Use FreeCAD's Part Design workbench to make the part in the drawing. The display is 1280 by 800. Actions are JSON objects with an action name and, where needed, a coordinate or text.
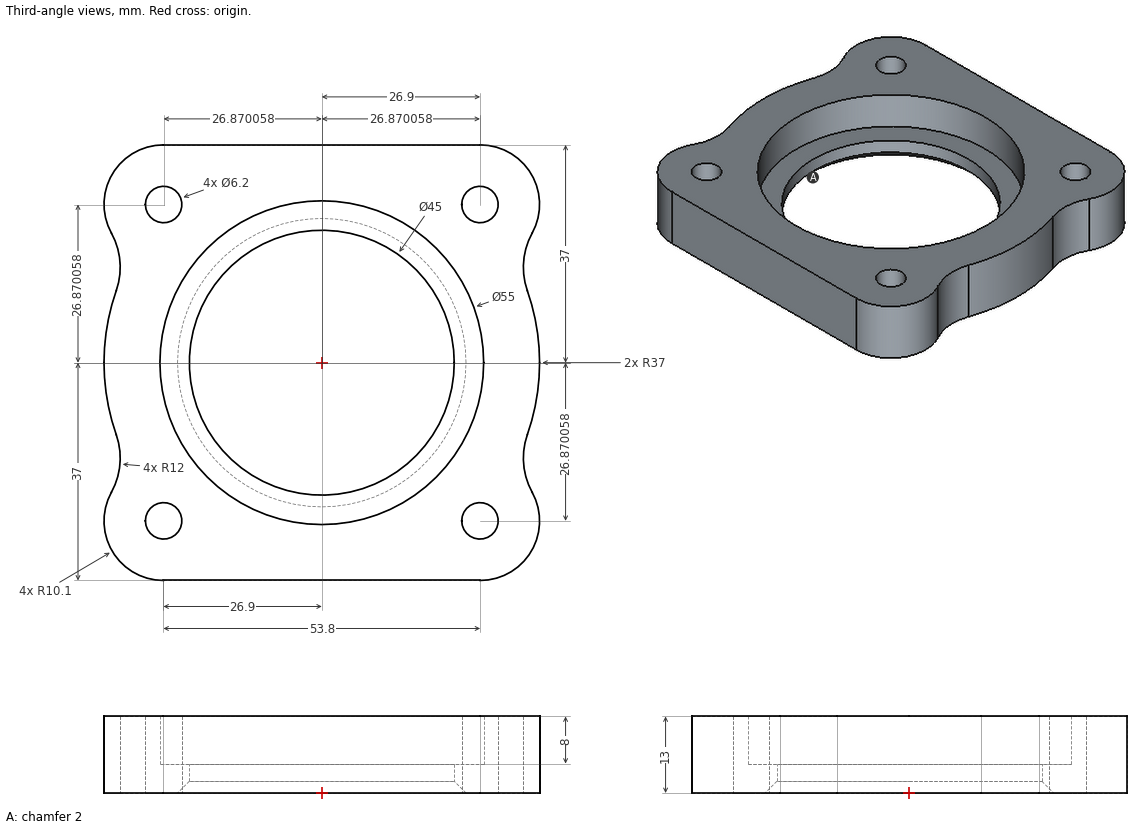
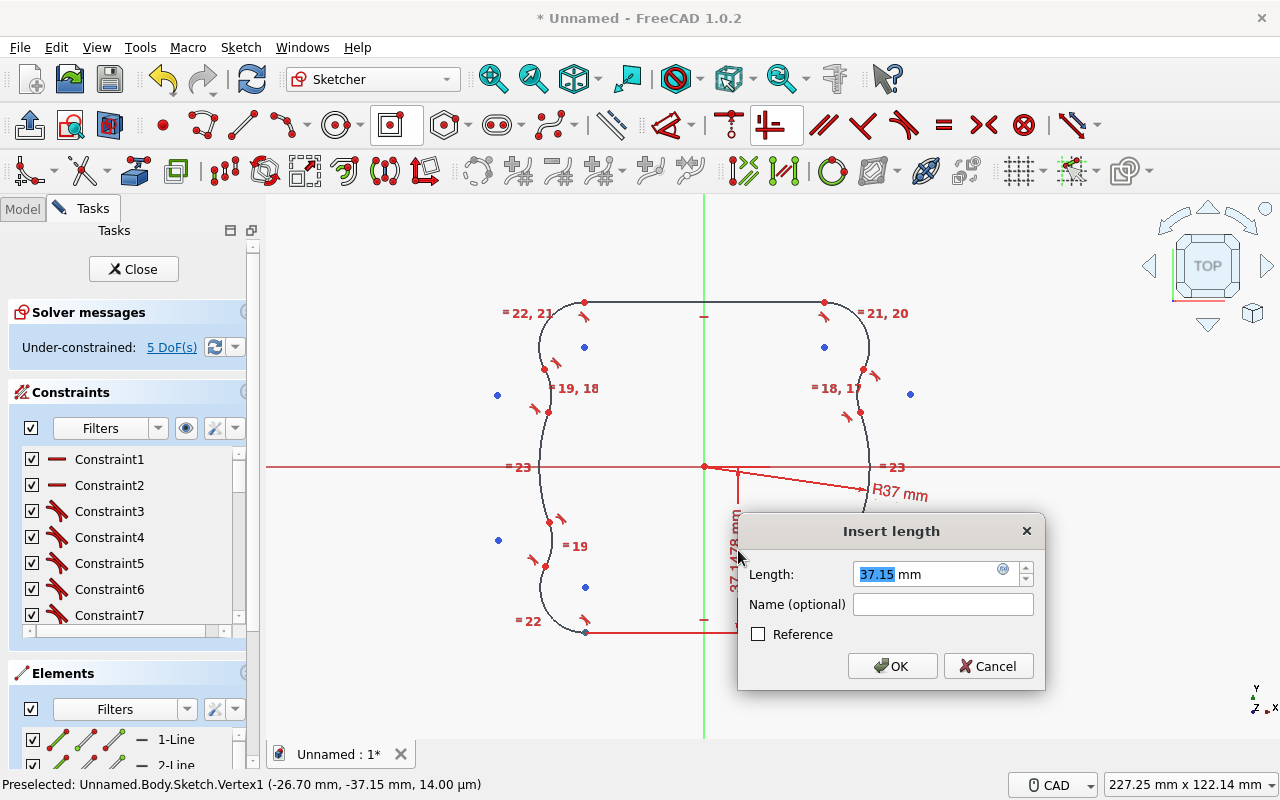
{"action": "type", "text": "37"}
{"action": "key", "text": "Return"}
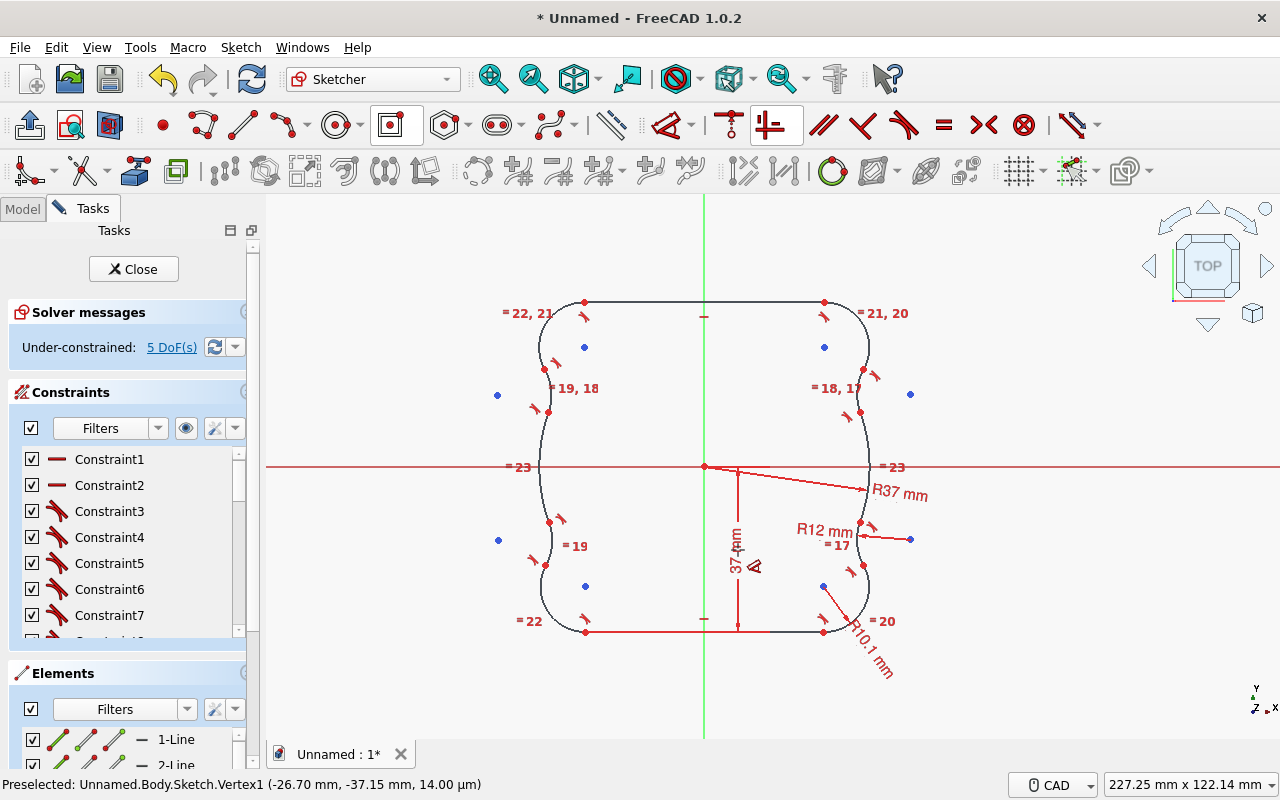
{"action": "left_click", "coordinate": [824, 302]}
{"action": "left_click", "coordinate": [670, 385]}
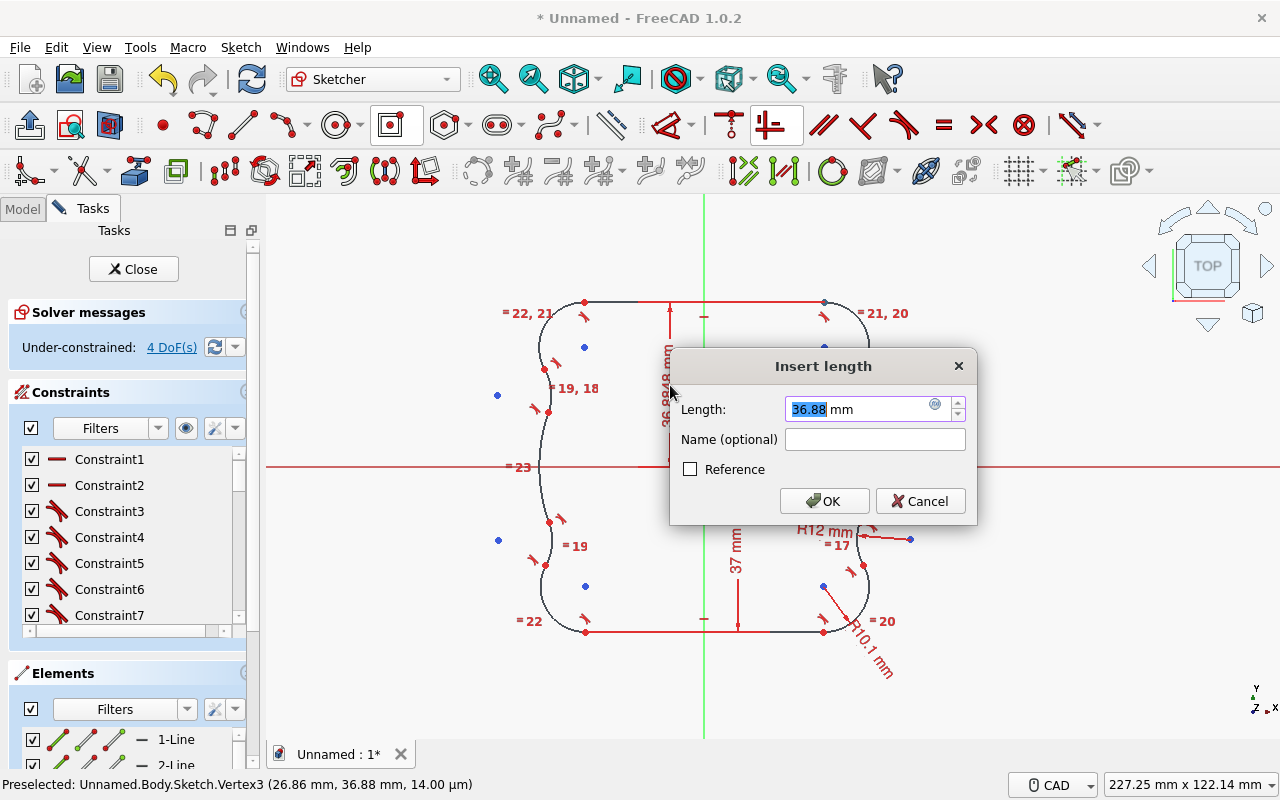
{"action": "type", "text": "37"}
{"action": "key", "text": "Return"}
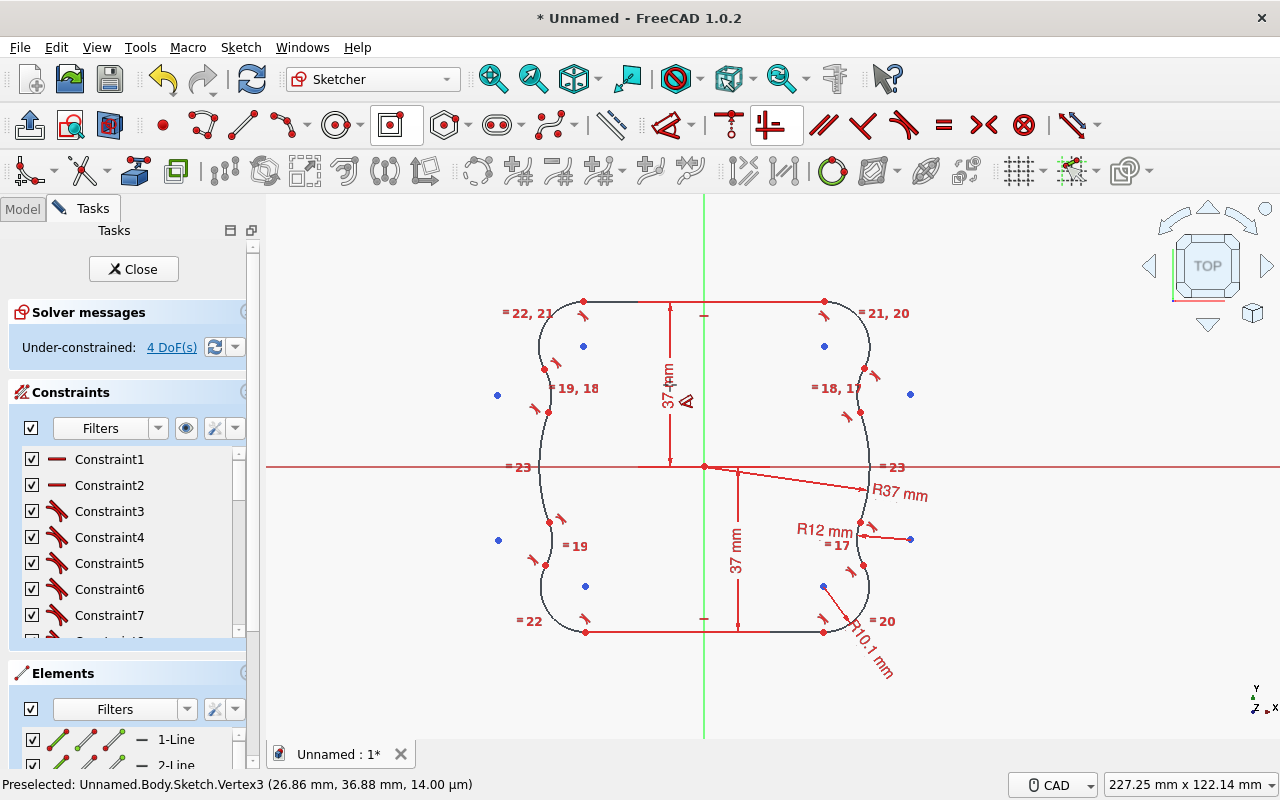
{"action": "left_click", "coordinate": [657, 632]}
{"action": "left_click", "coordinate": [650, 666]}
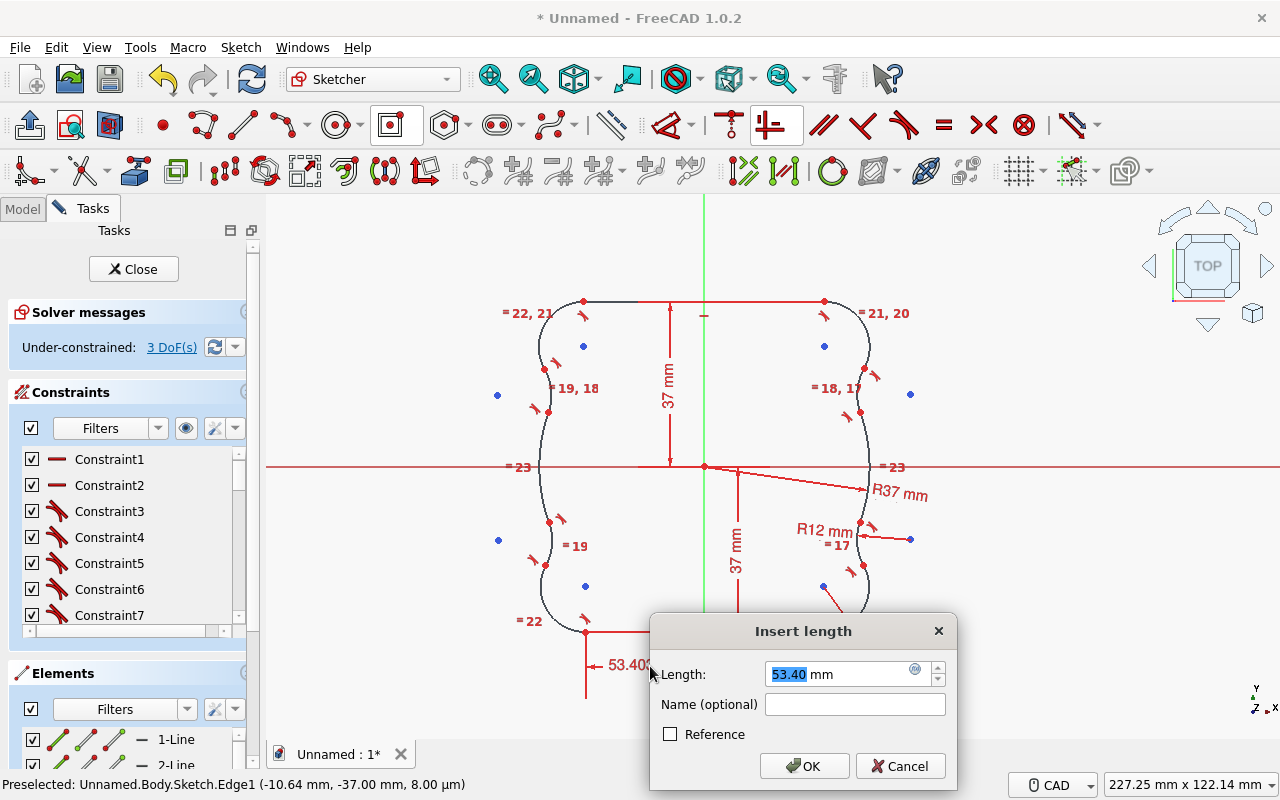
{"action": "type", "text": "53.8"}
{"action": "key", "text": "Return"}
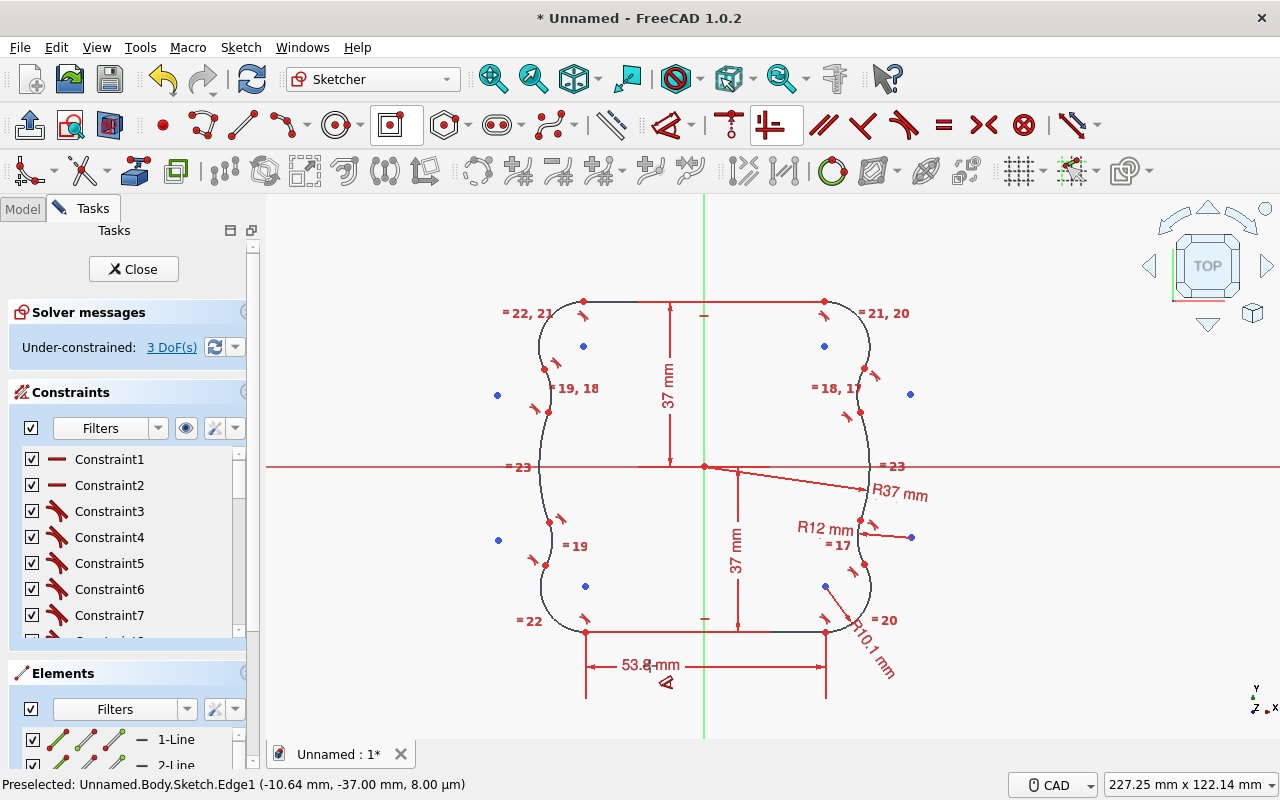
{"action": "left_click", "coordinate": [752, 302]}
{"action": "left_click", "coordinate": [649, 268]}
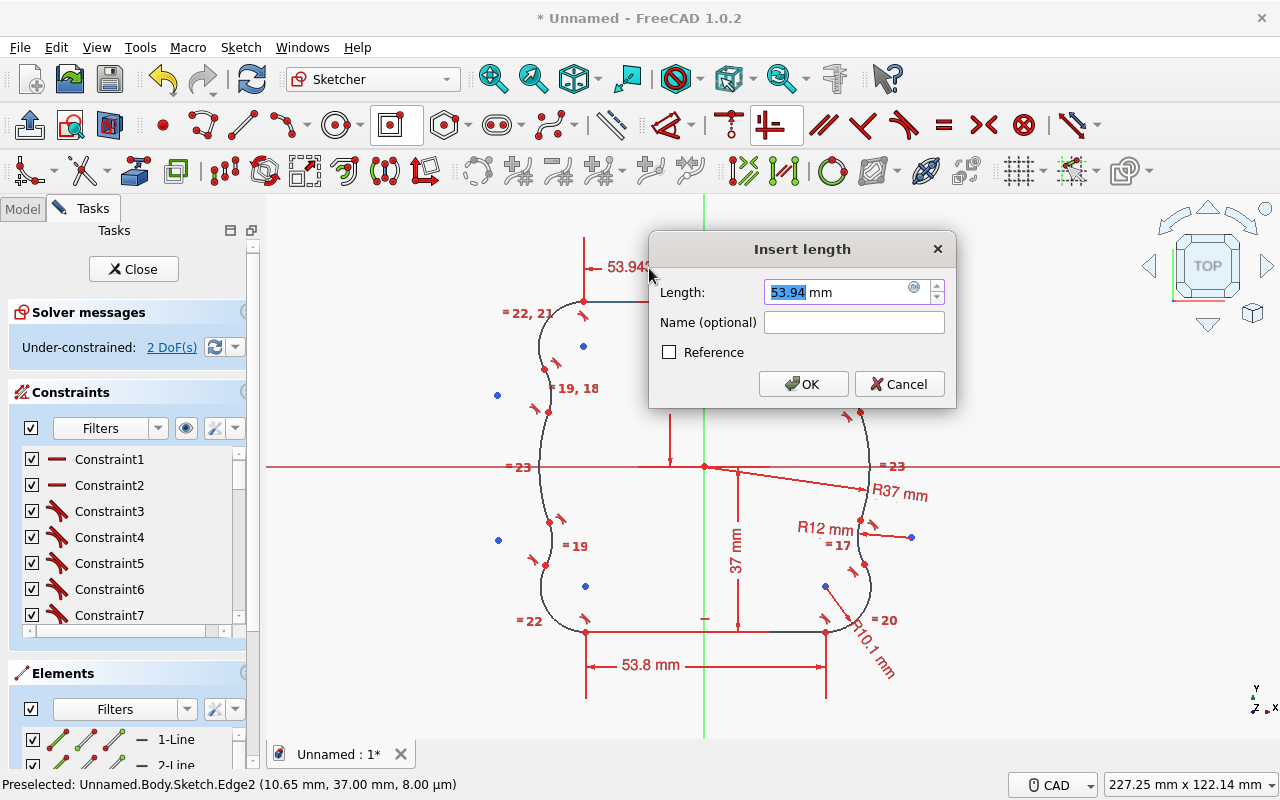
{"action": "type", "text": "53.8"}
{"action": "key", "text": "Return"}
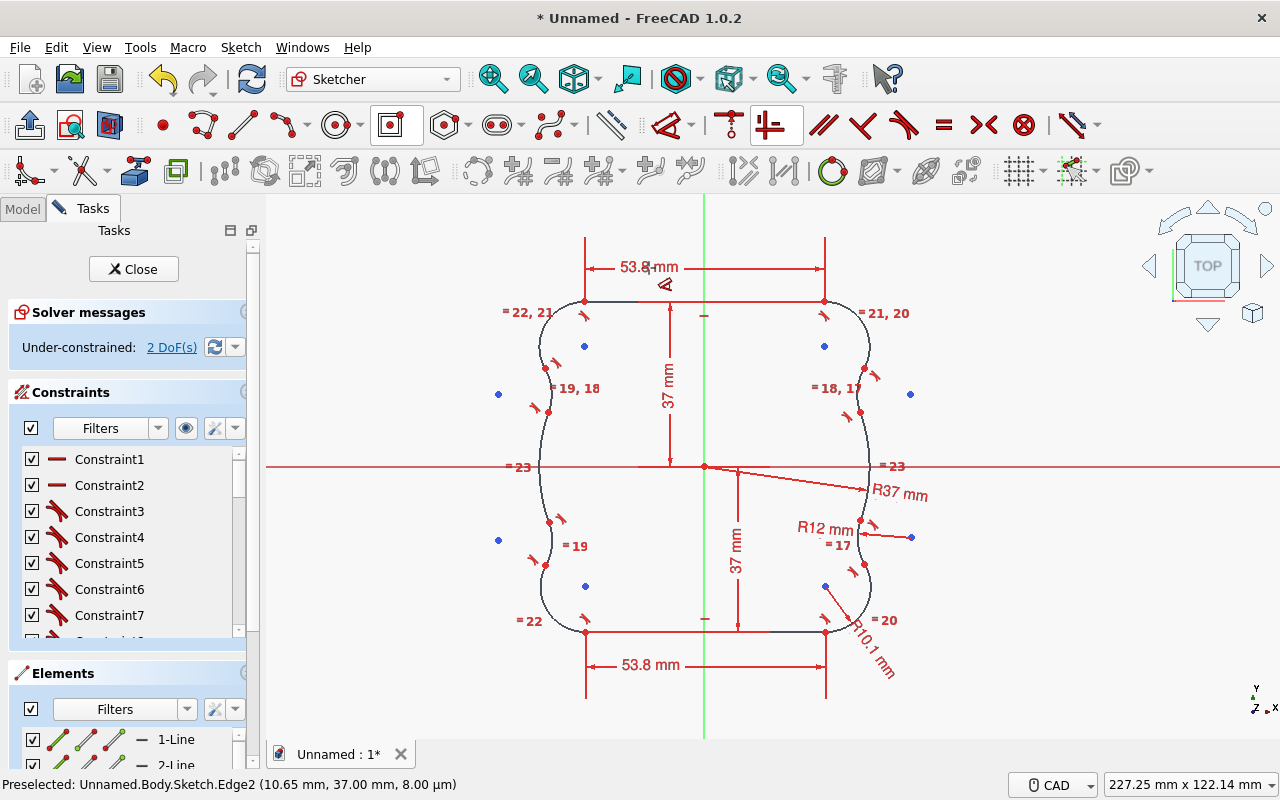
{"action": "left_click", "coordinate": [586, 632]}
{"action": "left_click", "coordinate": [645, 433]}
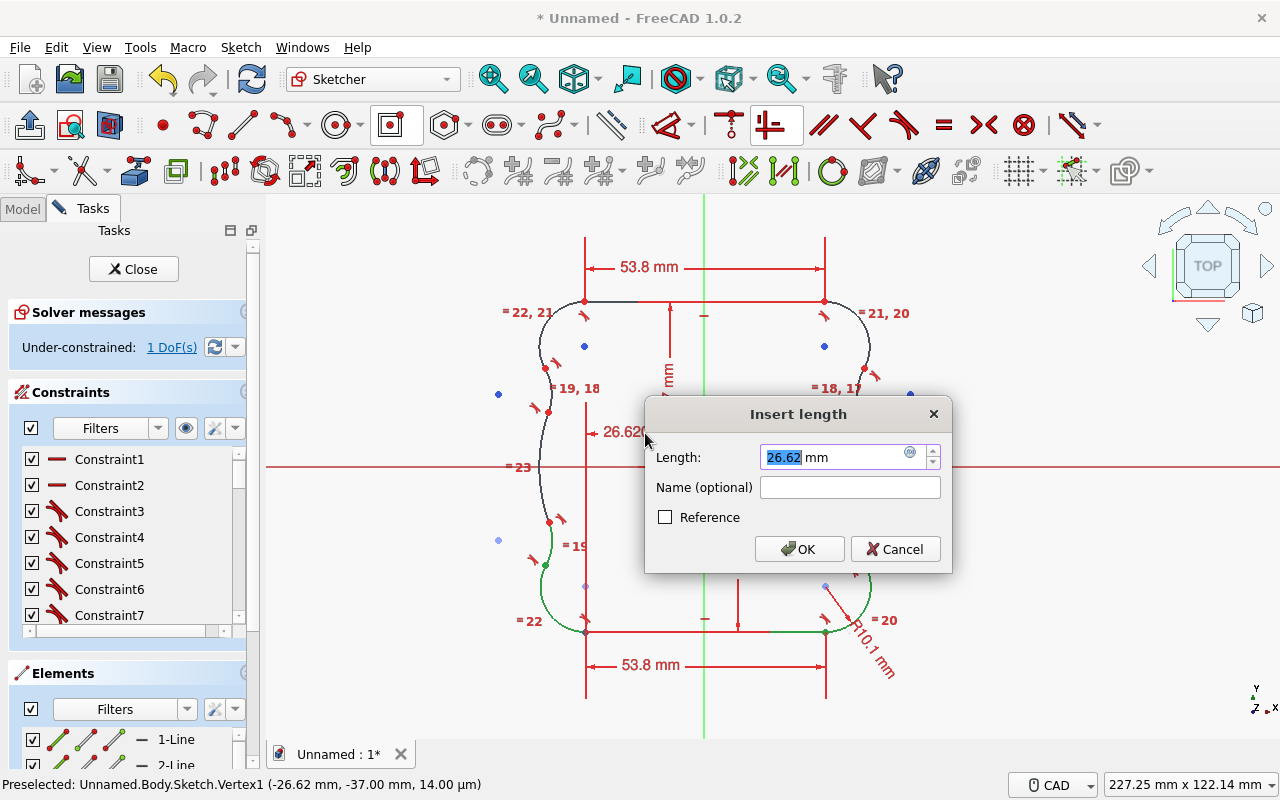
{"action": "type", "text": "26.9"}
{"action": "key", "text": "Return"}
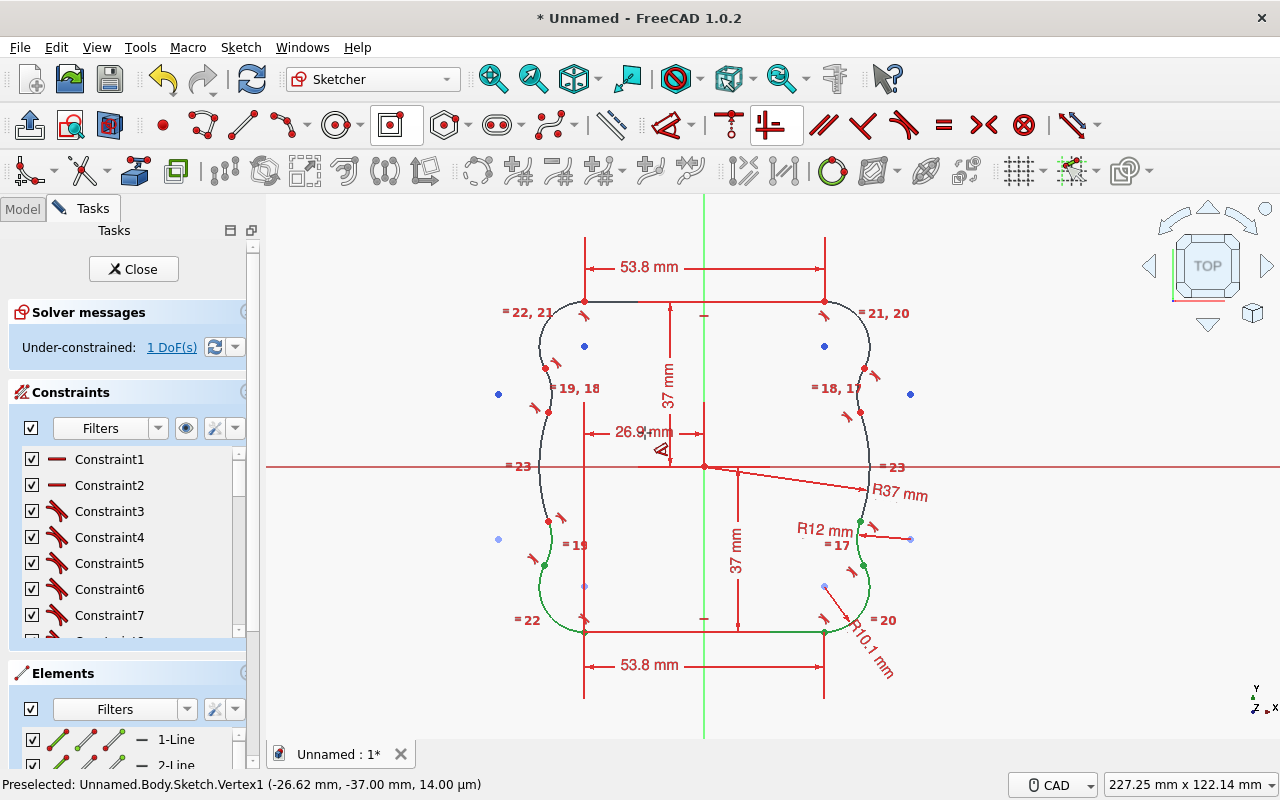
{"action": "left_click", "coordinate": [825, 302]}
{"action": "left_click", "coordinate": [765, 268]}